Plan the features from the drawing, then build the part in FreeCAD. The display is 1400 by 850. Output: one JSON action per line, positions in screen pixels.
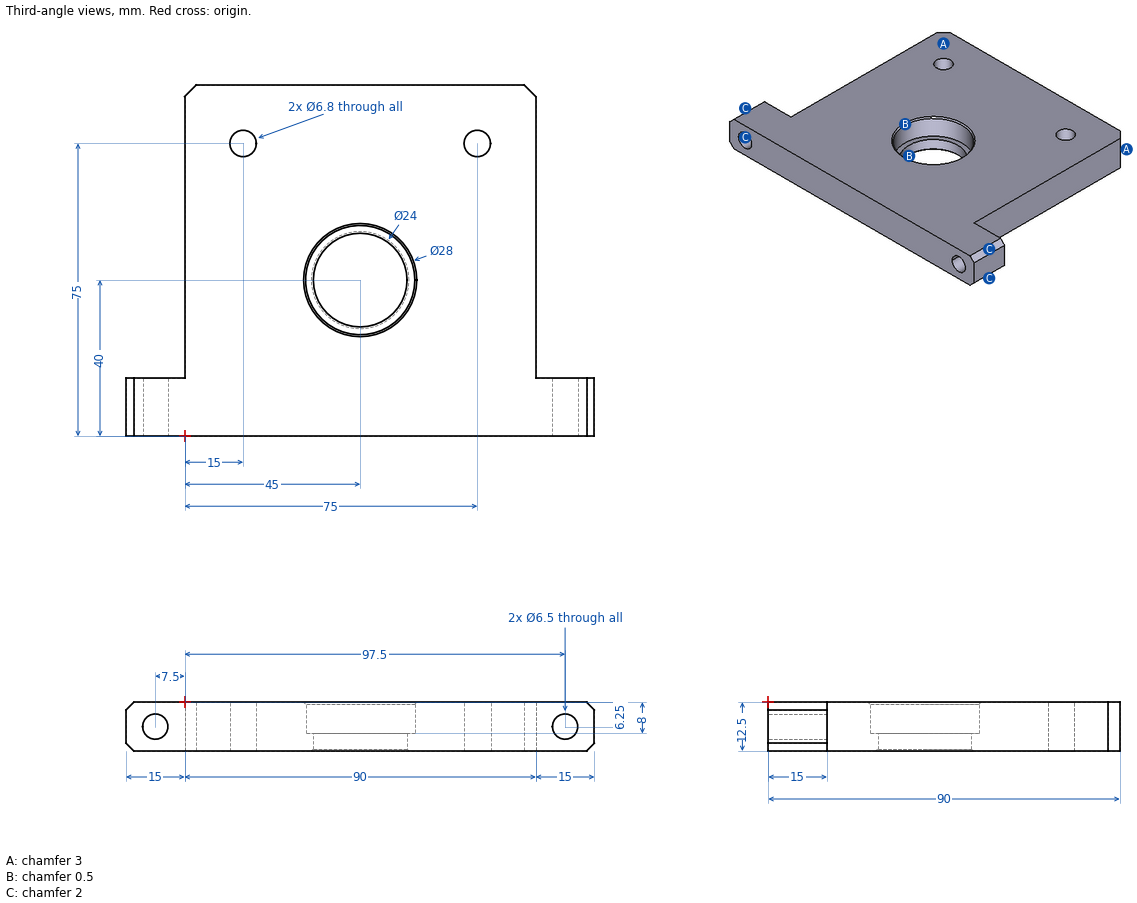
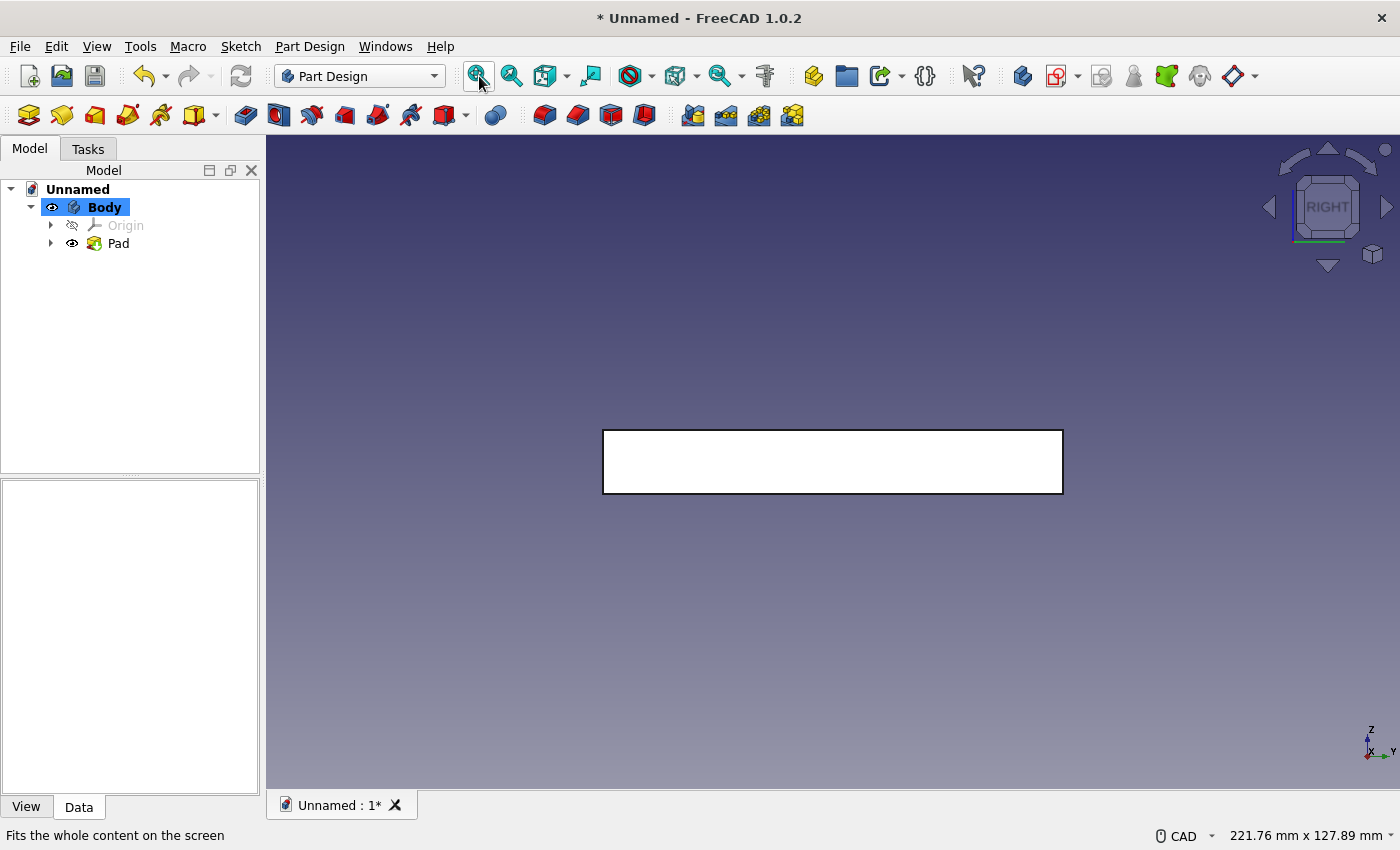
{"action": "left_click", "coordinate": [479, 76]}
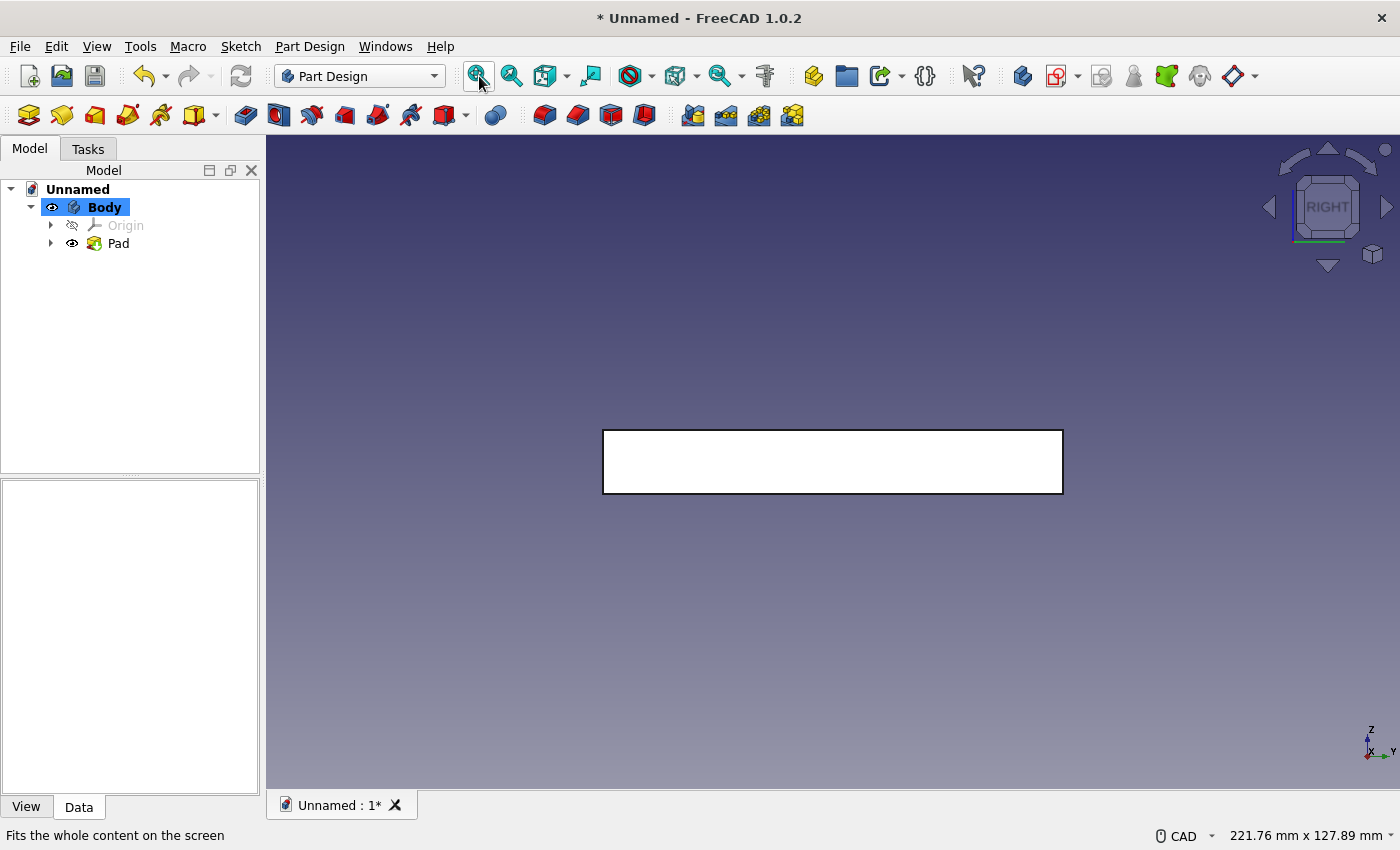
{"action": "left_click", "coordinate": [1063, 461]}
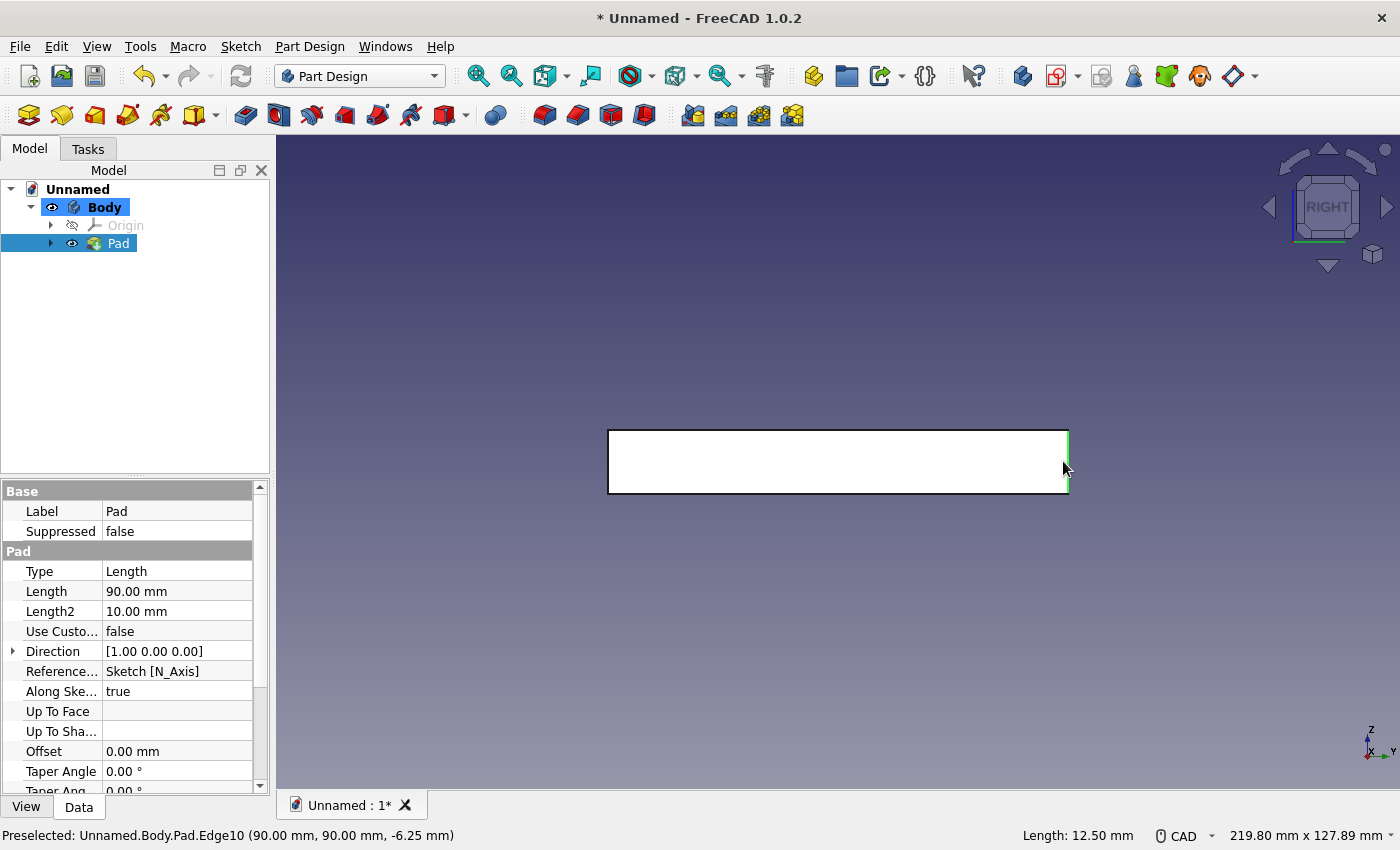
{"action": "key", "text": "5"}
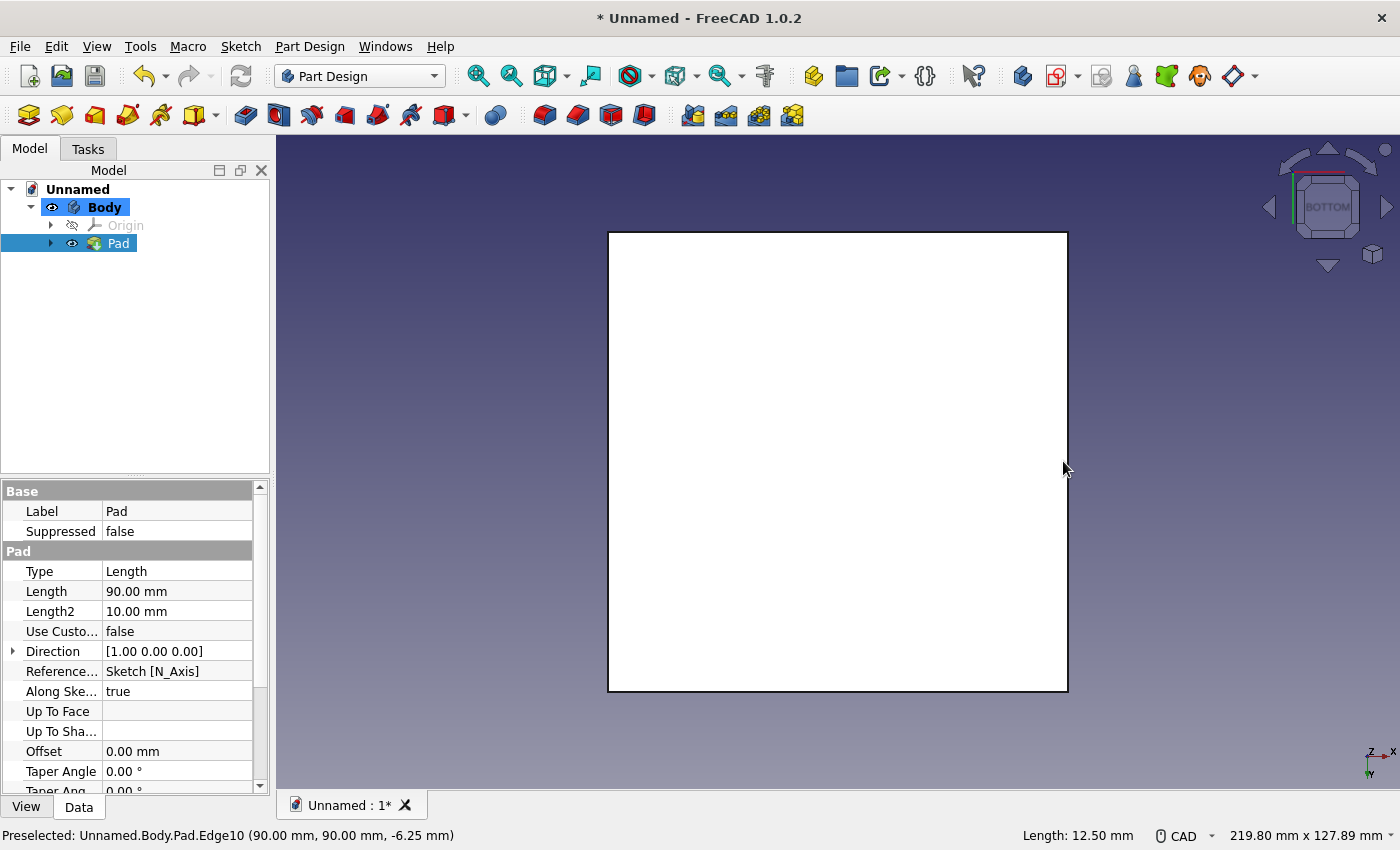
{"action": "key", "text": "4"}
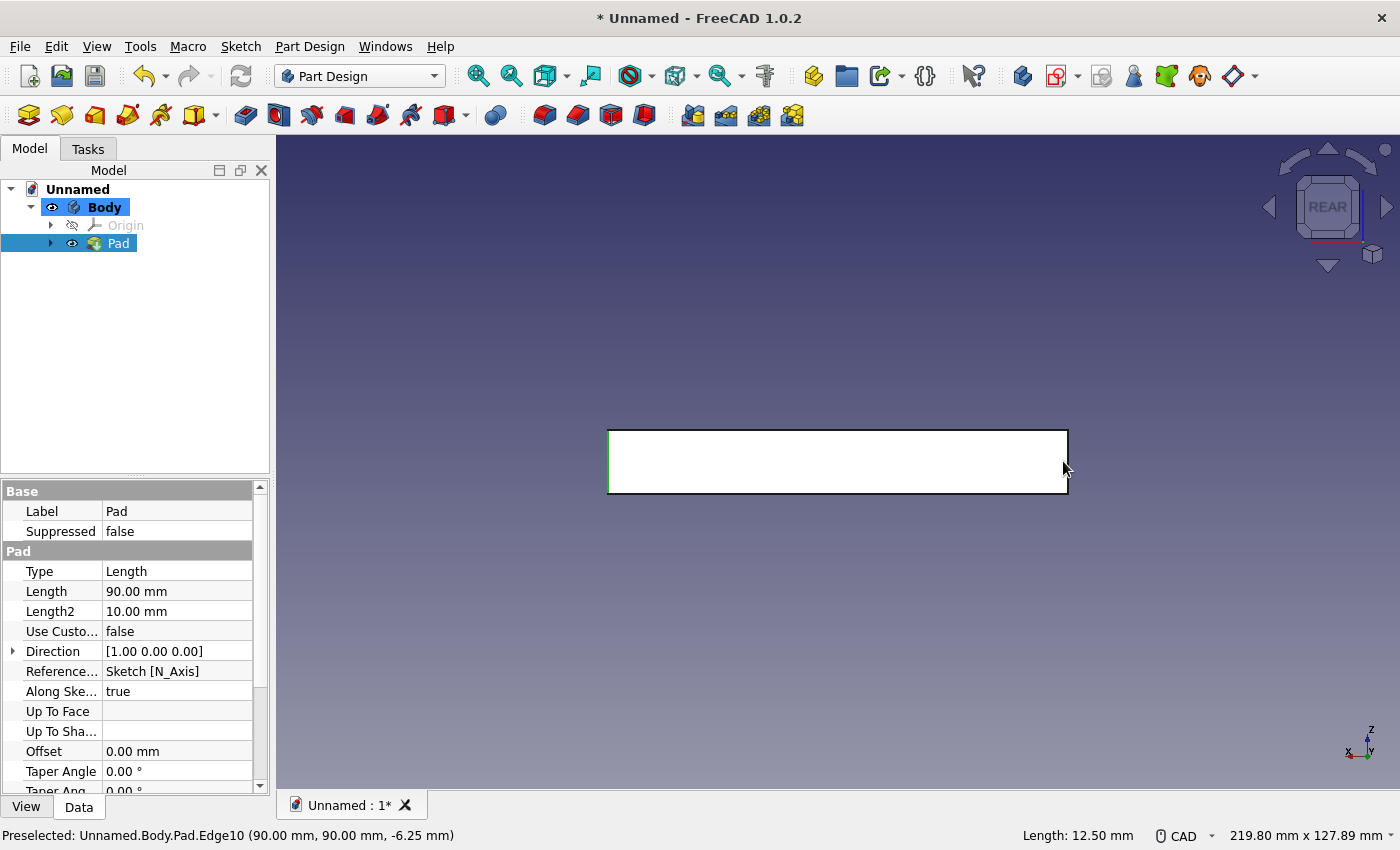
{"action": "left_click", "coordinate": [479, 76]}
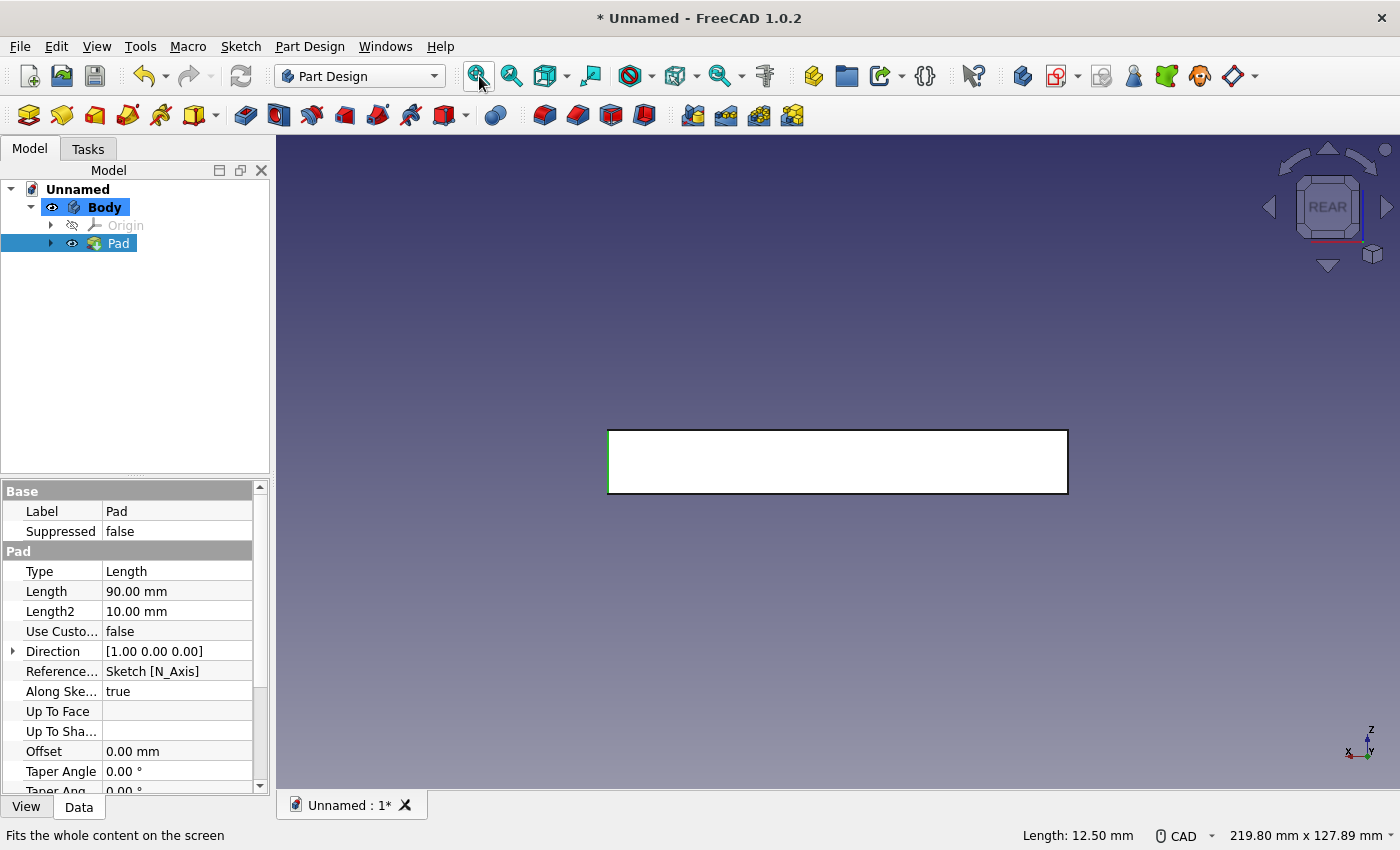
{"action": "left_click", "coordinate": [1068, 461], "text": "ctrl"}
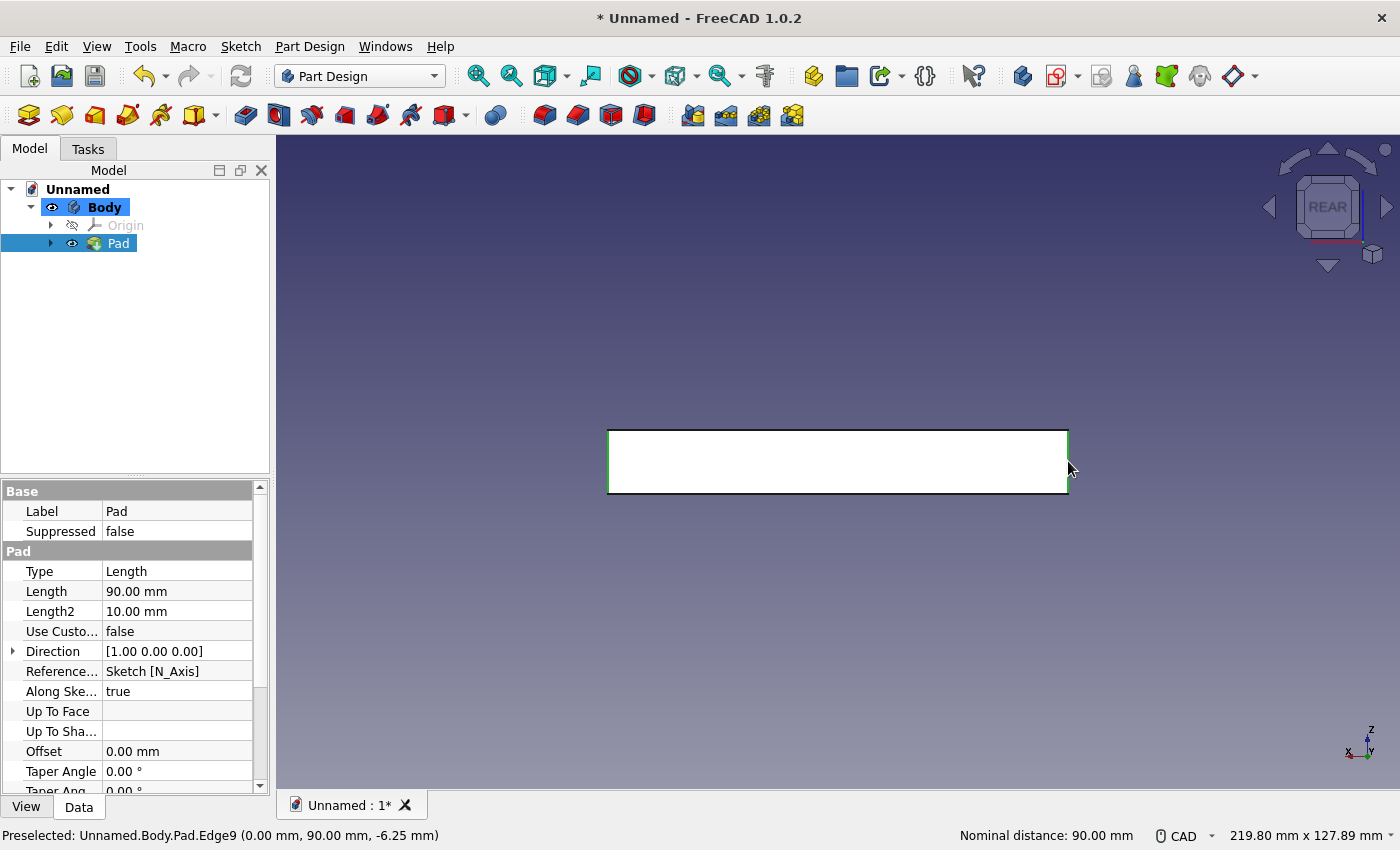
{"action": "left_click", "coordinate": [578, 116]}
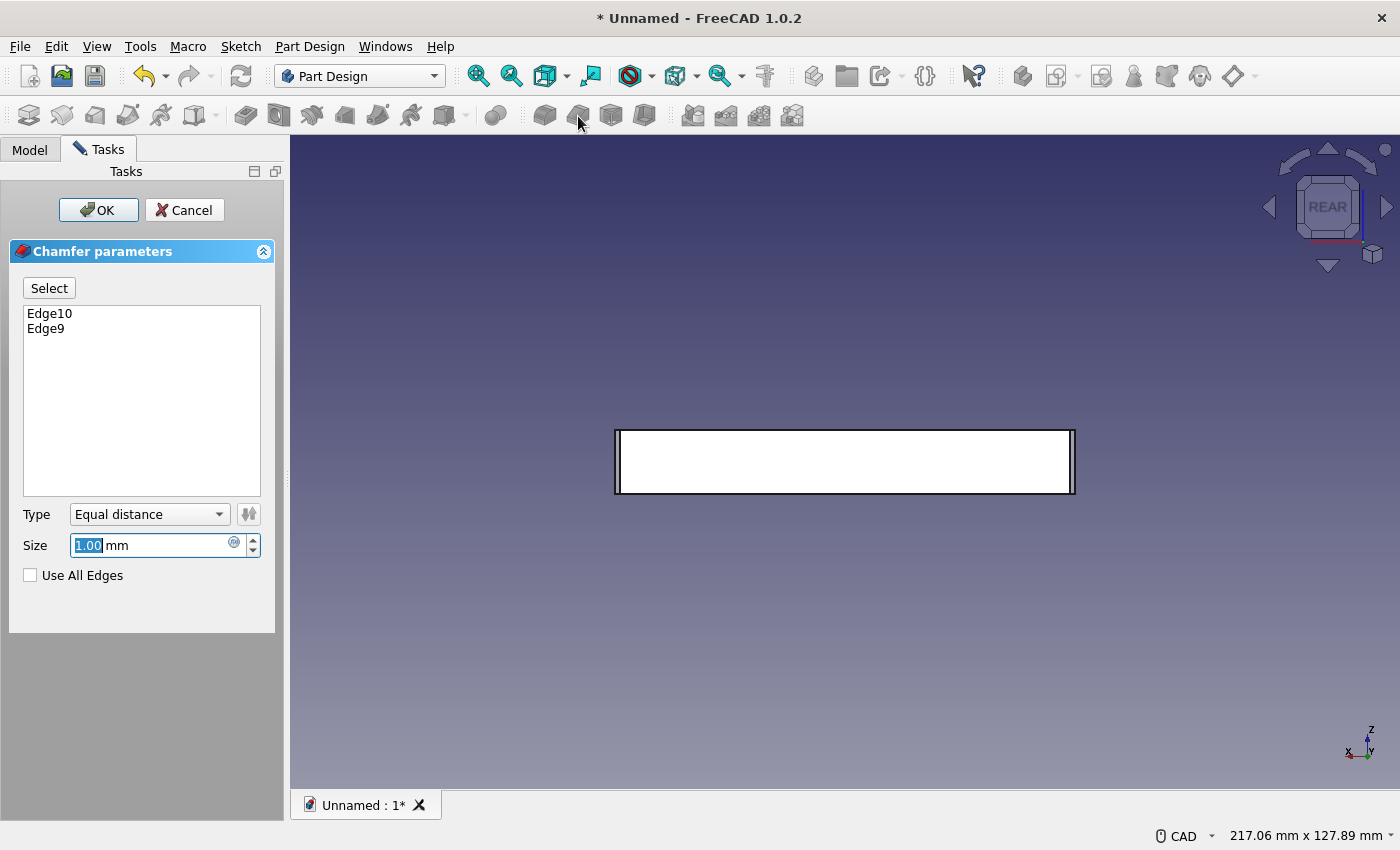
{"action": "type", "text": "3"}
{"action": "key", "text": "Tab"}